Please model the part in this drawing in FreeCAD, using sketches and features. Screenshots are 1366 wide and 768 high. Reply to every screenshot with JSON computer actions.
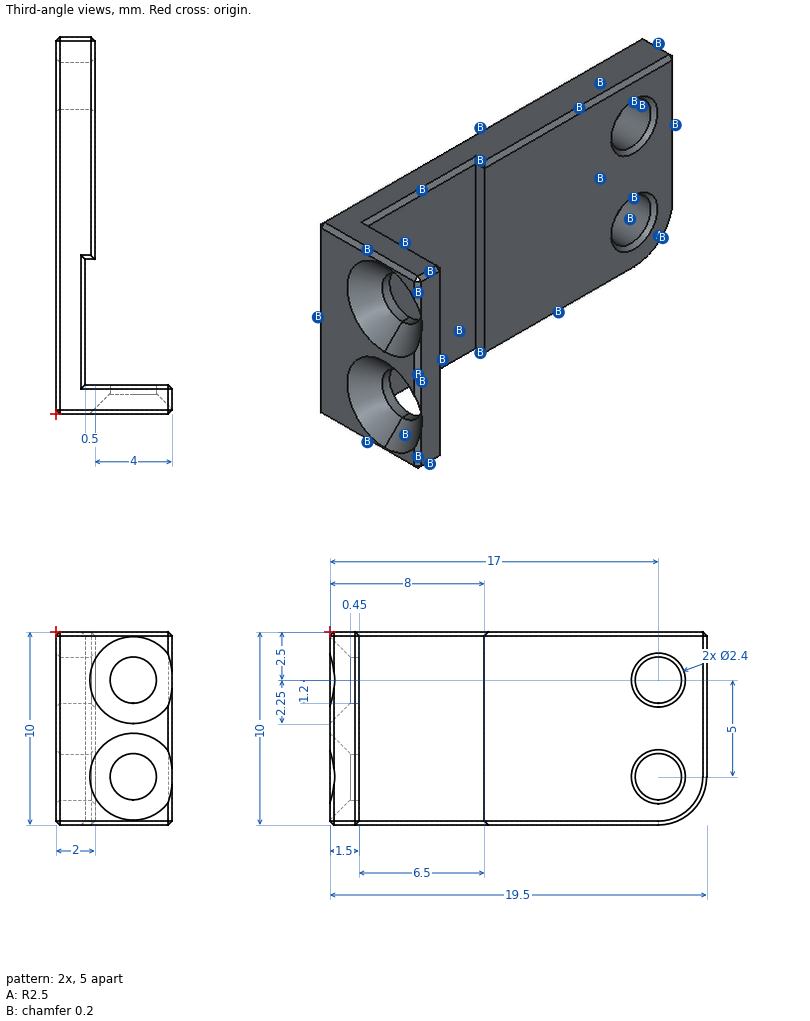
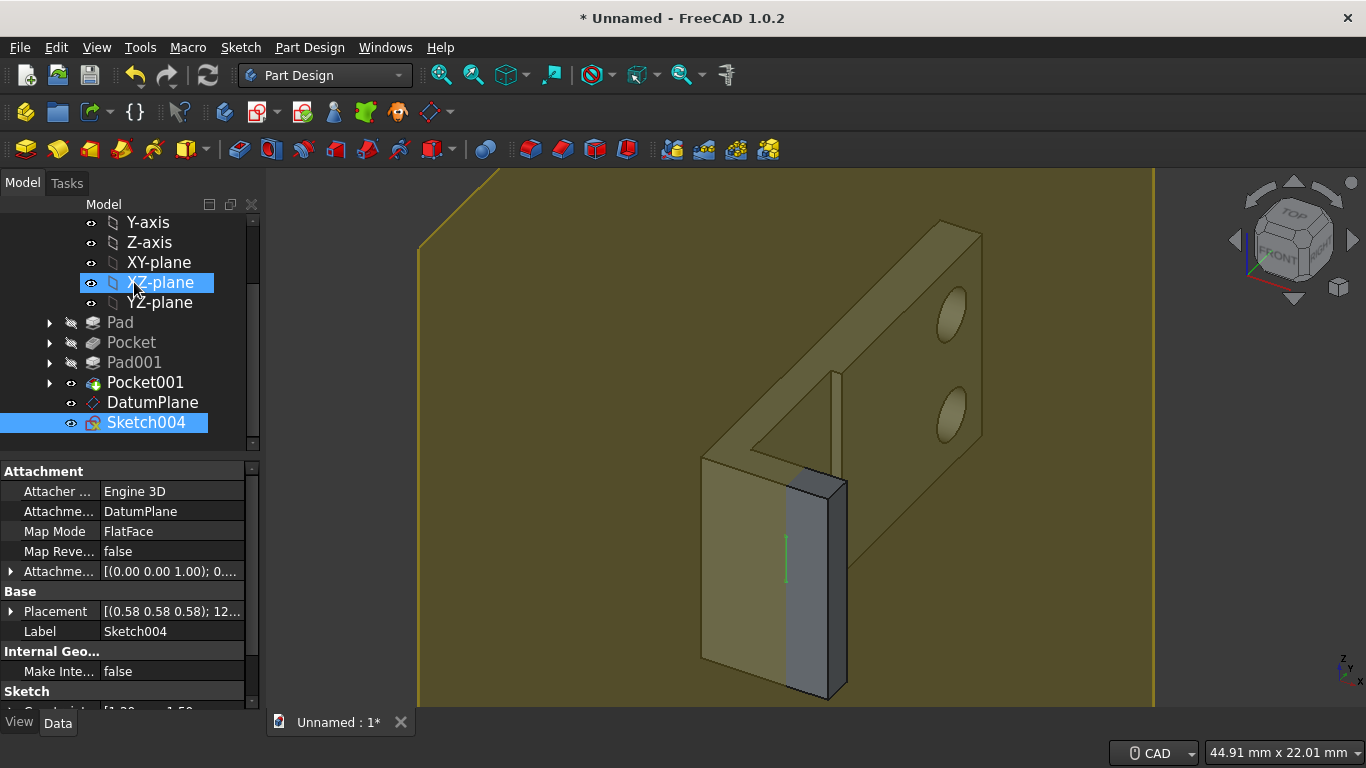
{"action": "left_click", "coordinate": [304, 150]}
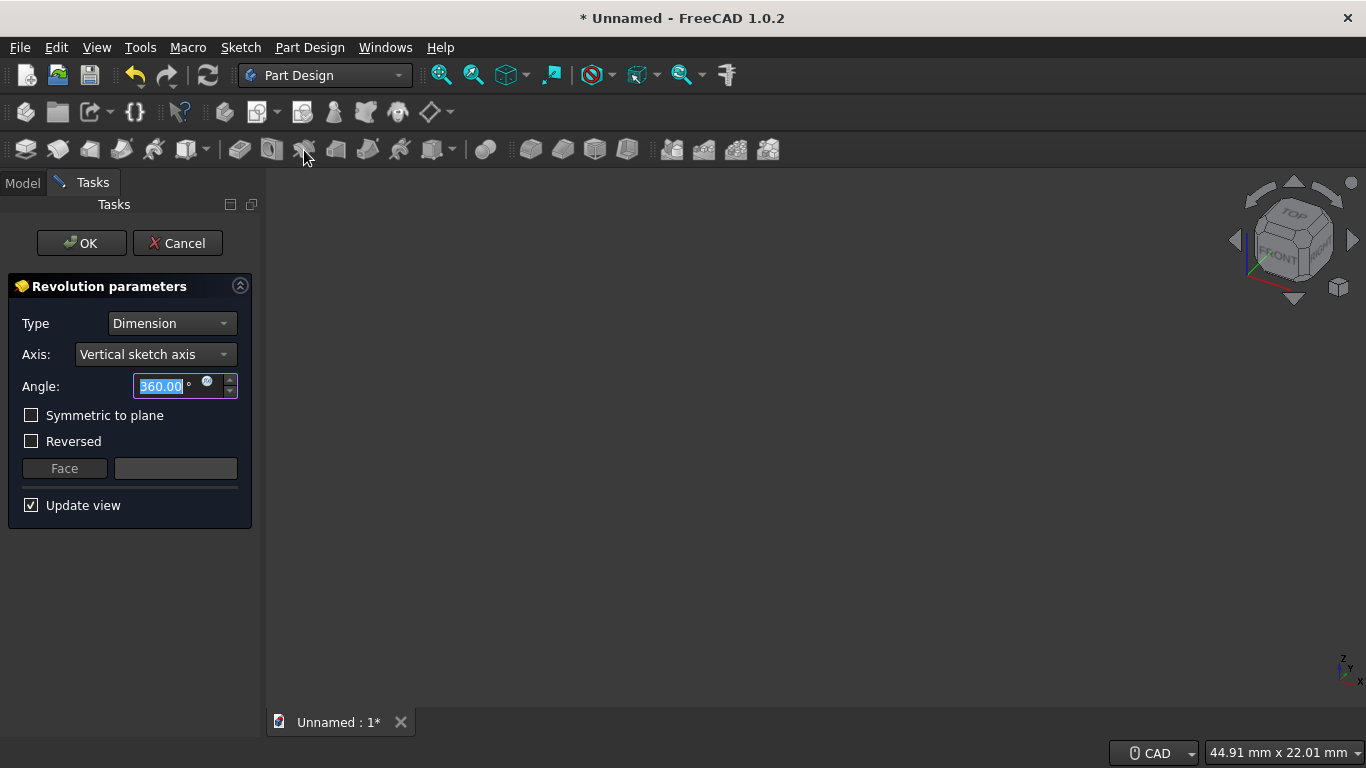
{"action": "left_click", "coordinate": [156, 354]}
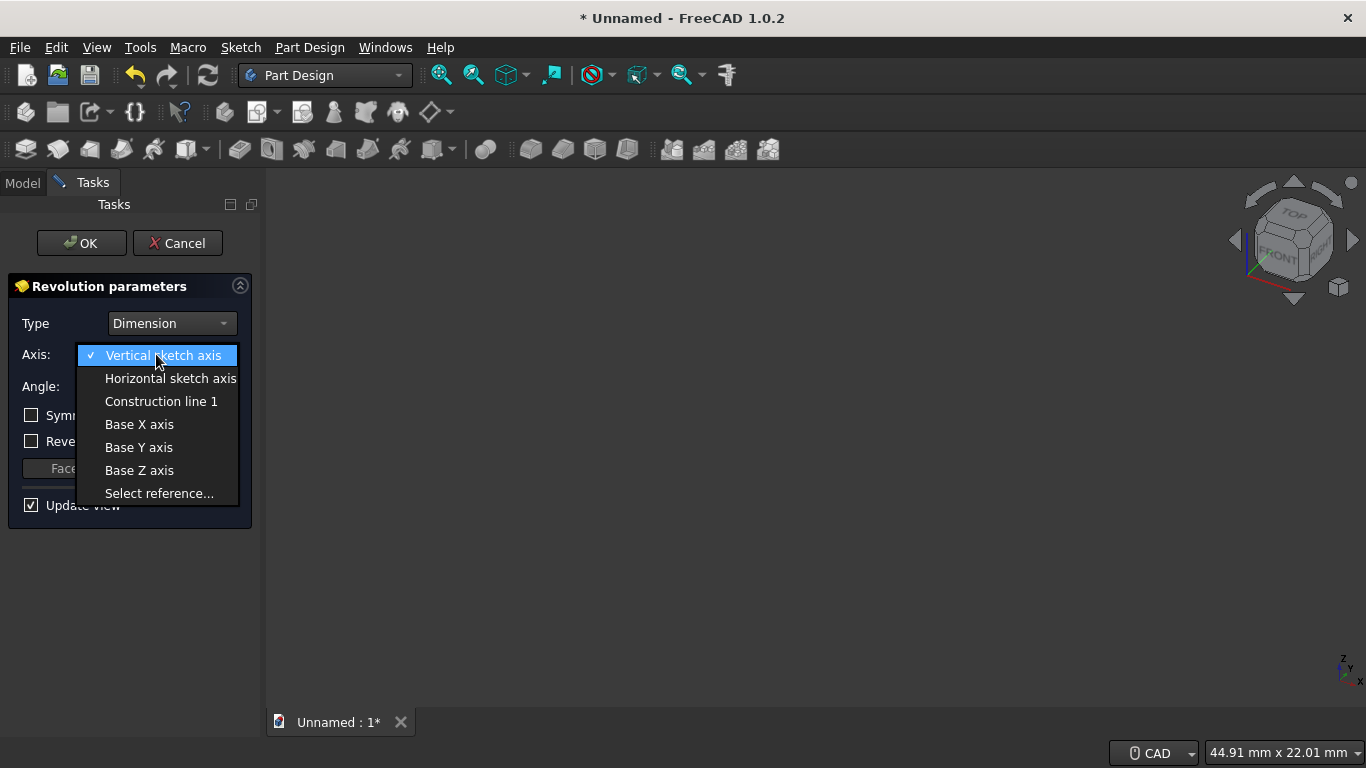
{"action": "left_click", "coordinate": [156, 402]}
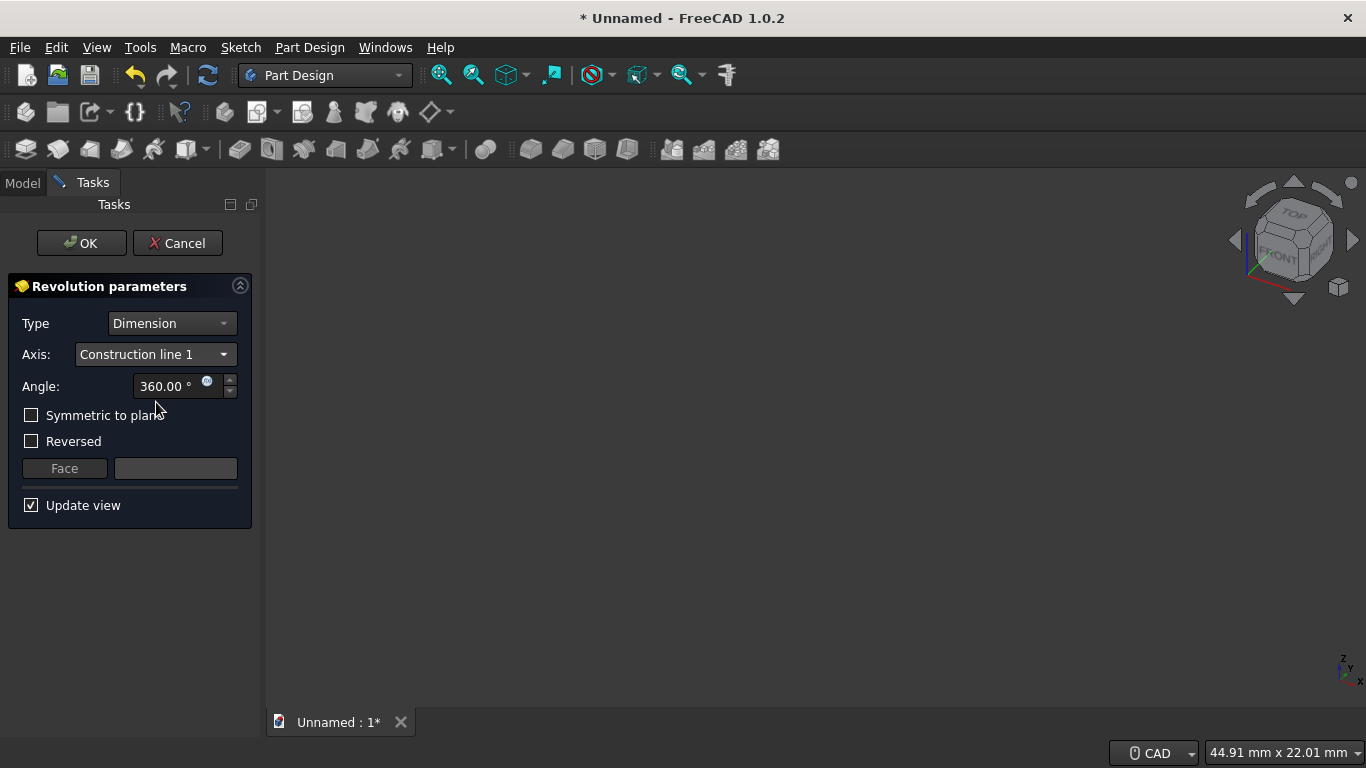
{"action": "left_click", "coordinate": [82, 243]}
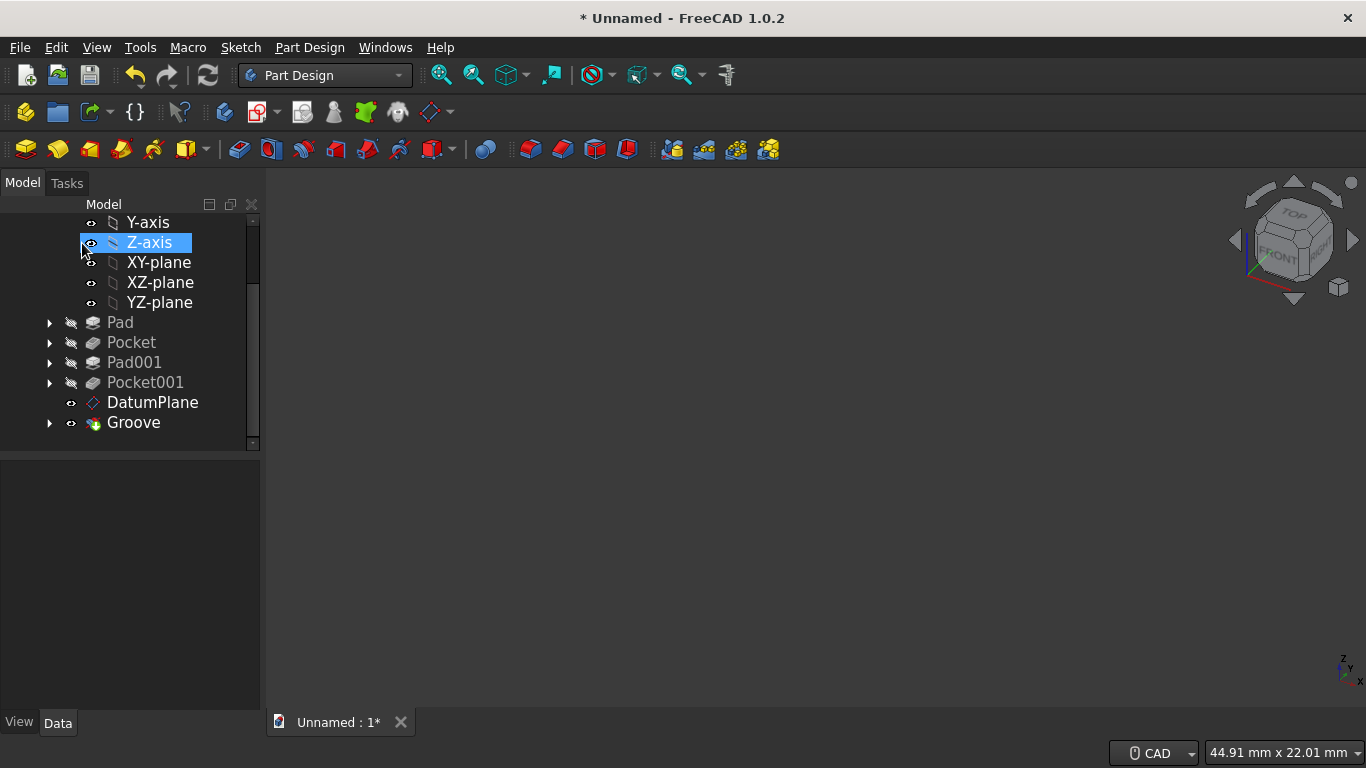
{"action": "left_click", "coordinate": [116, 403]}
{"action": "key", "text": "space"}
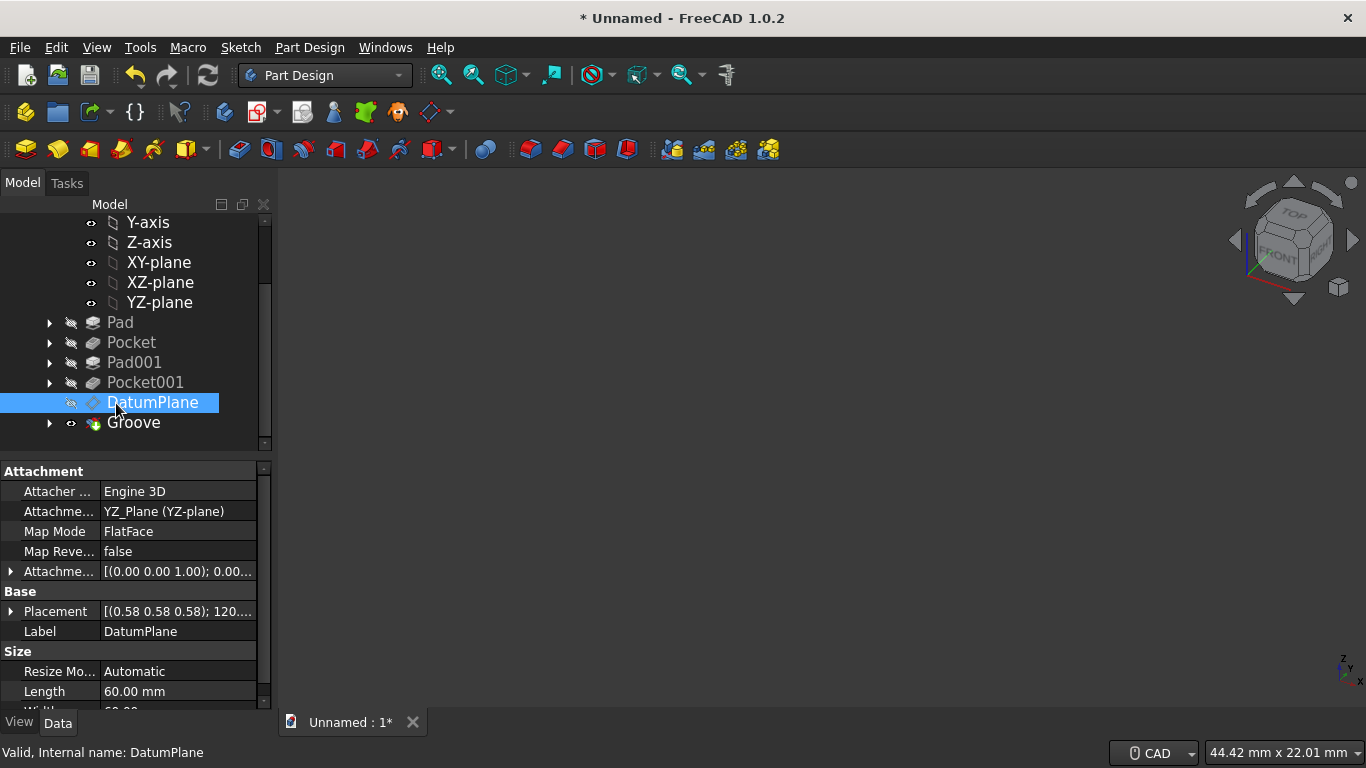
{"action": "left_click", "coordinate": [442, 76]}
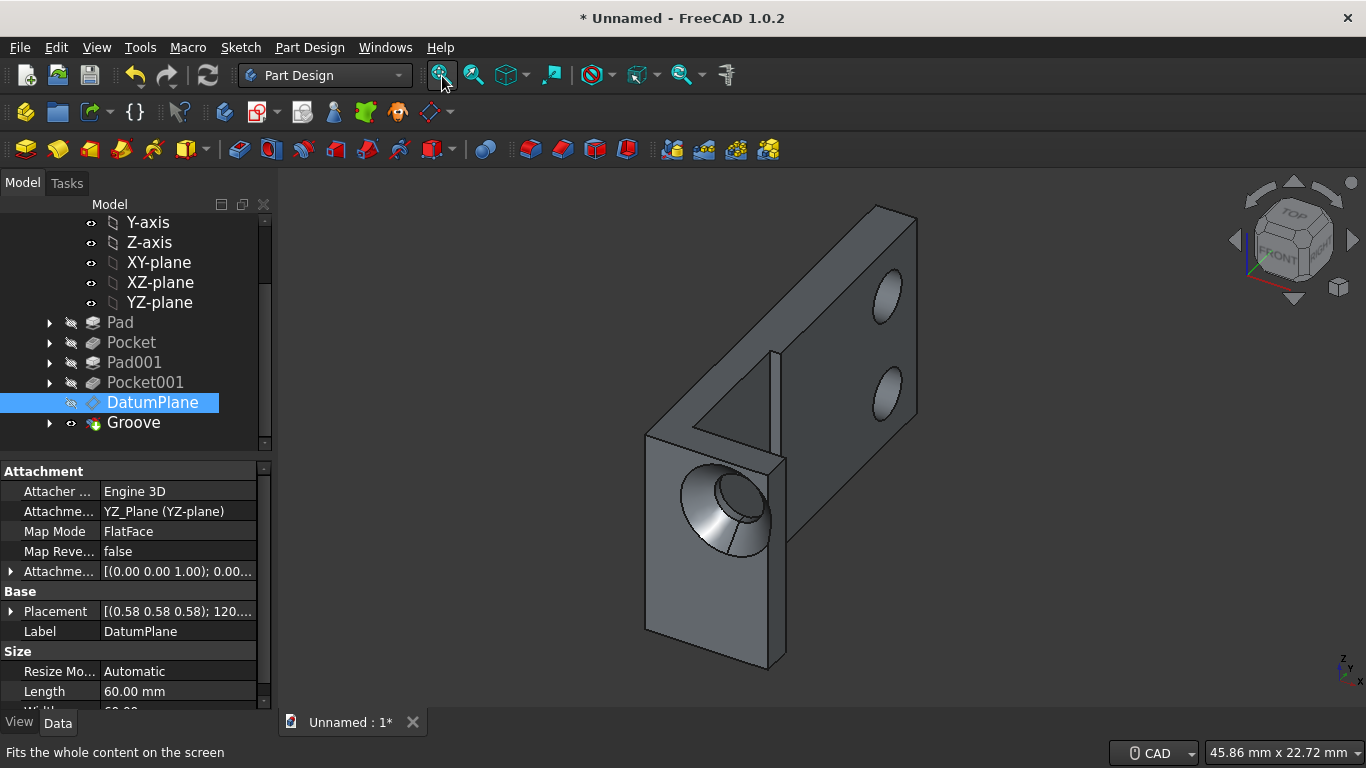
{"action": "left_click", "coordinate": [116, 423]}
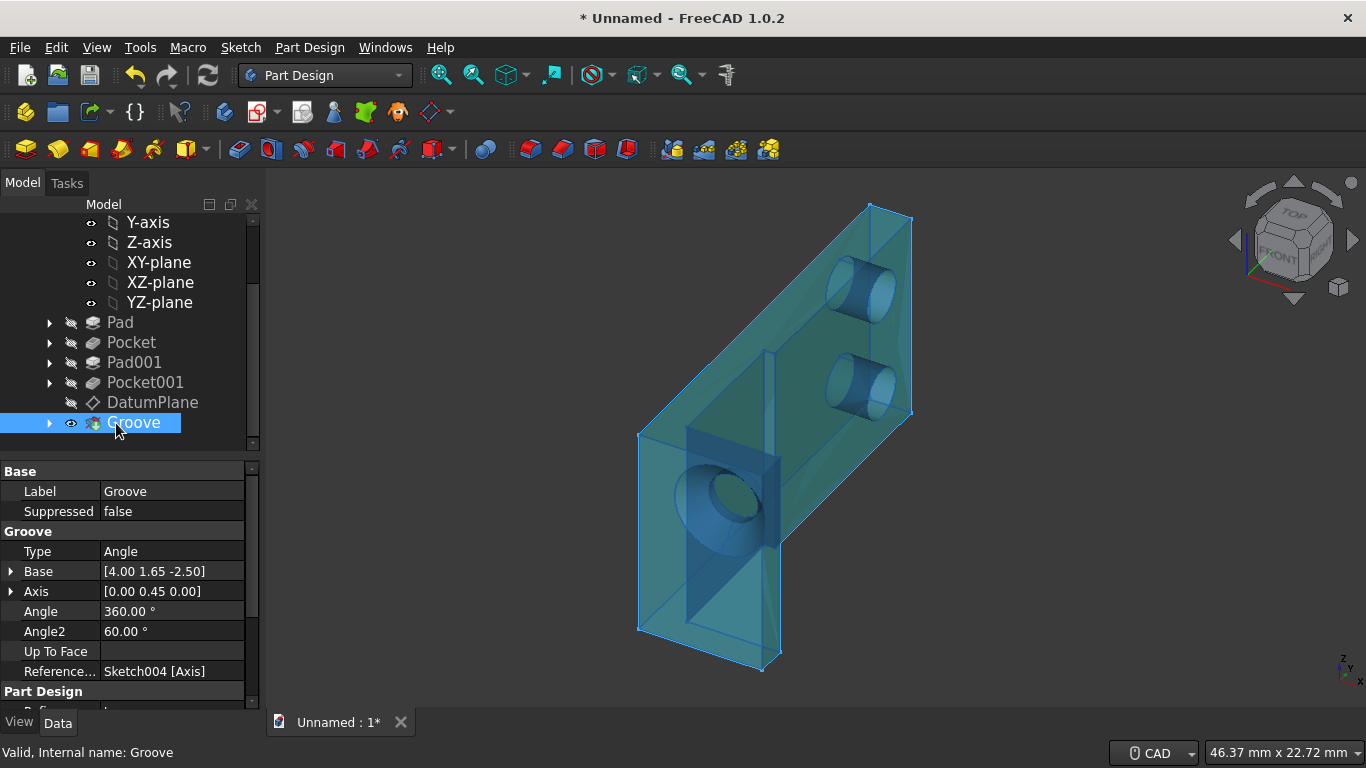
{"action": "left_click", "coordinate": [704, 150]}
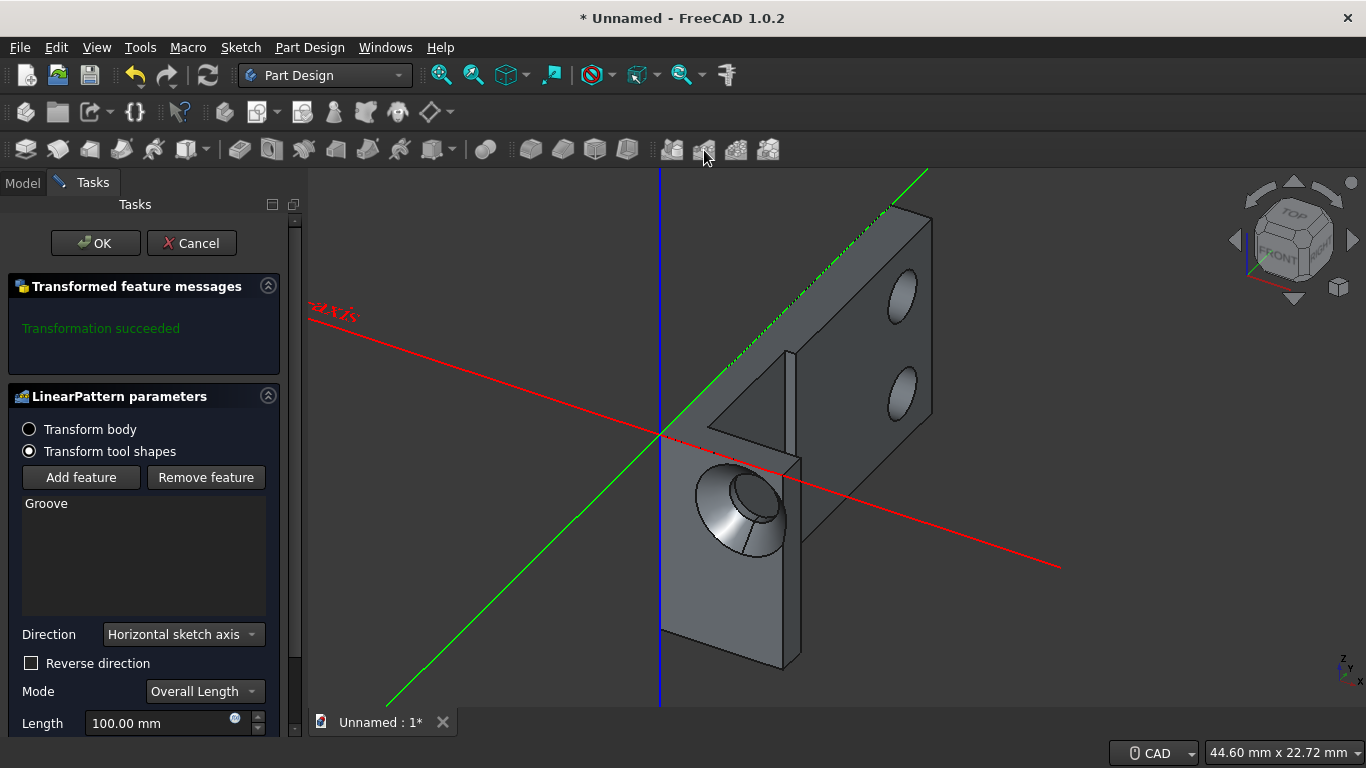
{"action": "left_click", "coordinate": [184, 634]}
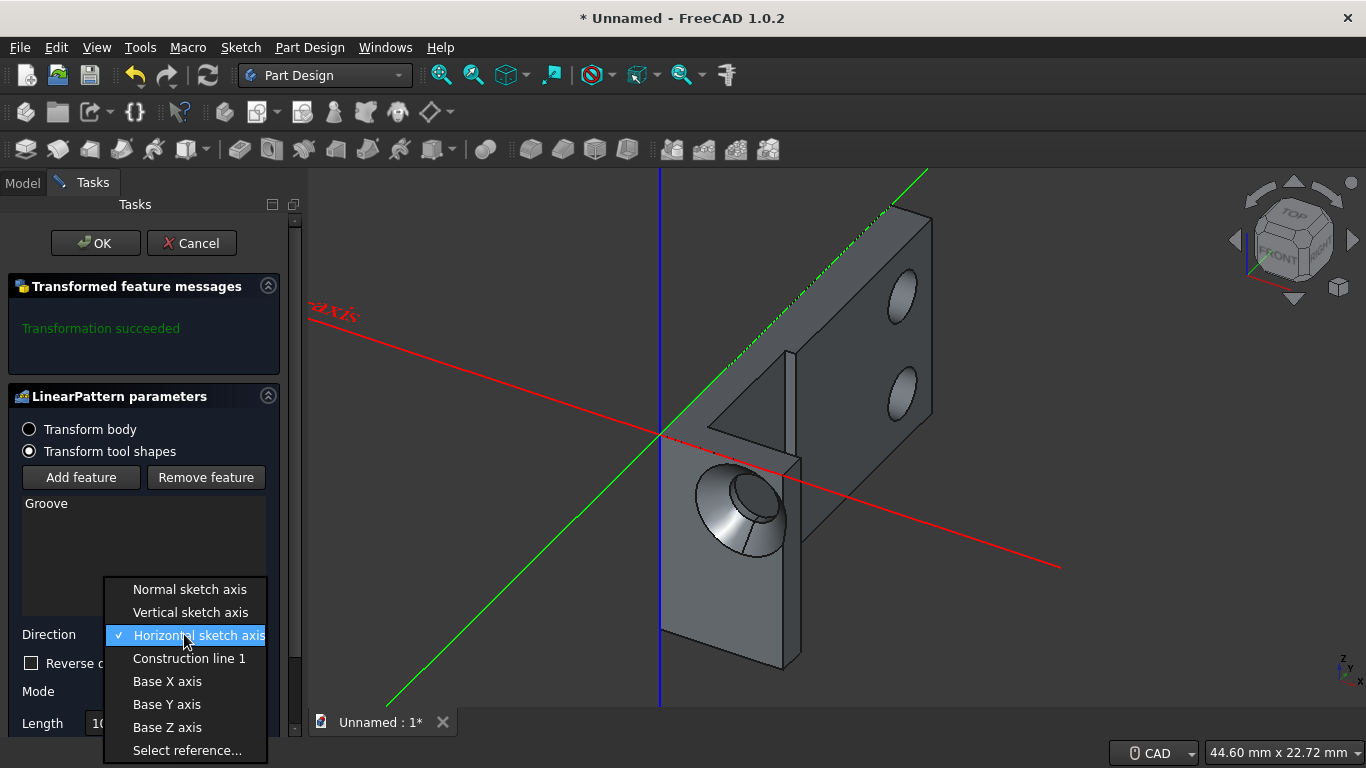
{"action": "left_click", "coordinate": [184, 728]}